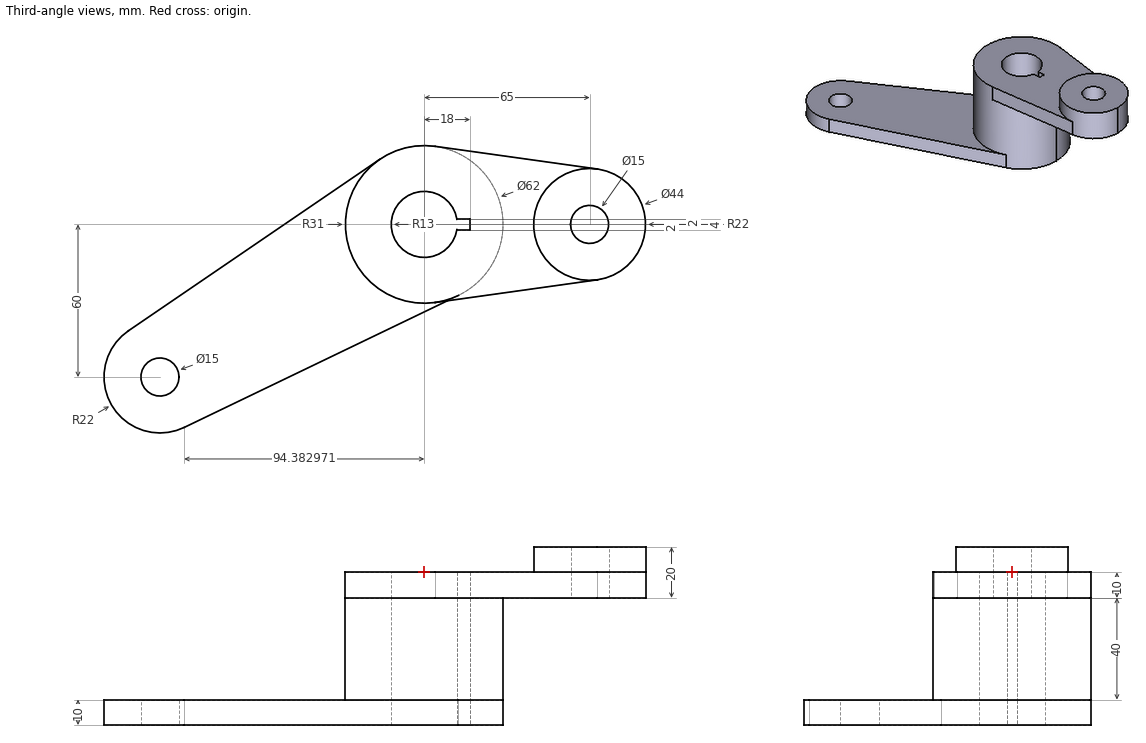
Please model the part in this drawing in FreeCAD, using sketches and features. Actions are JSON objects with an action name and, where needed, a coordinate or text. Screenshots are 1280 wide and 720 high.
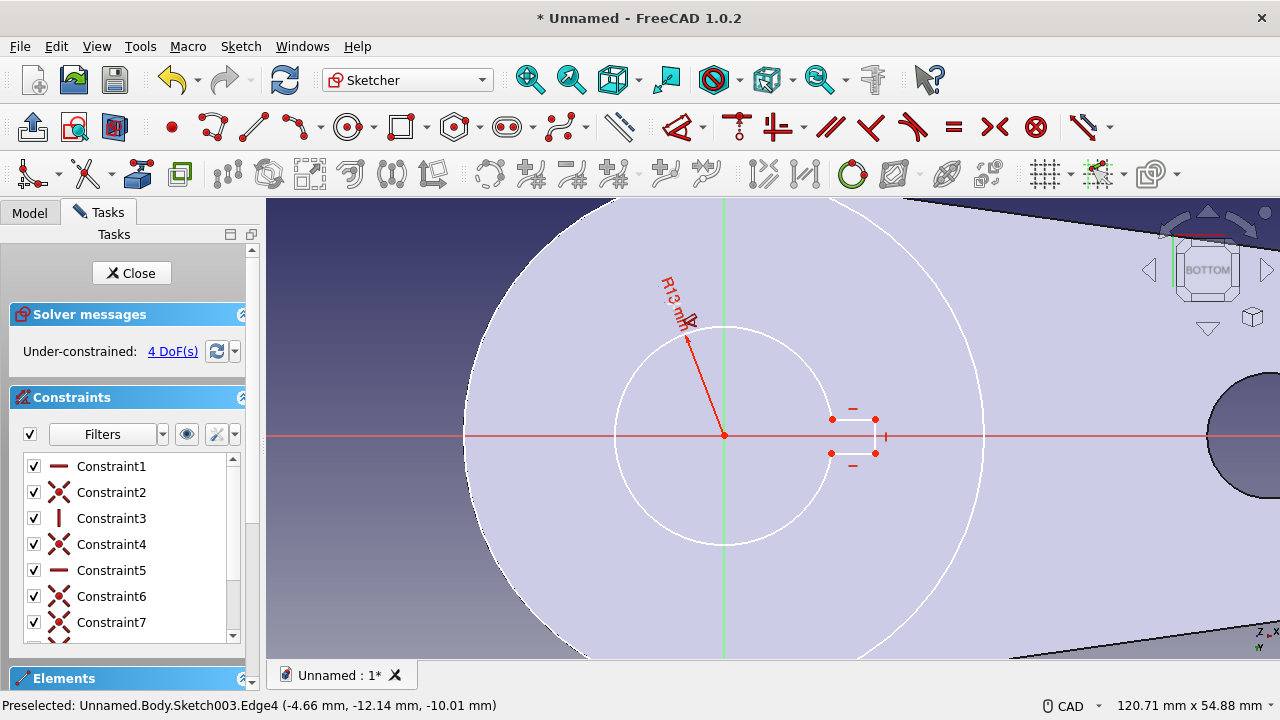
{"action": "left_click", "coordinate": [907, 251]}
{"action": "left_click", "coordinate": [930, 228]}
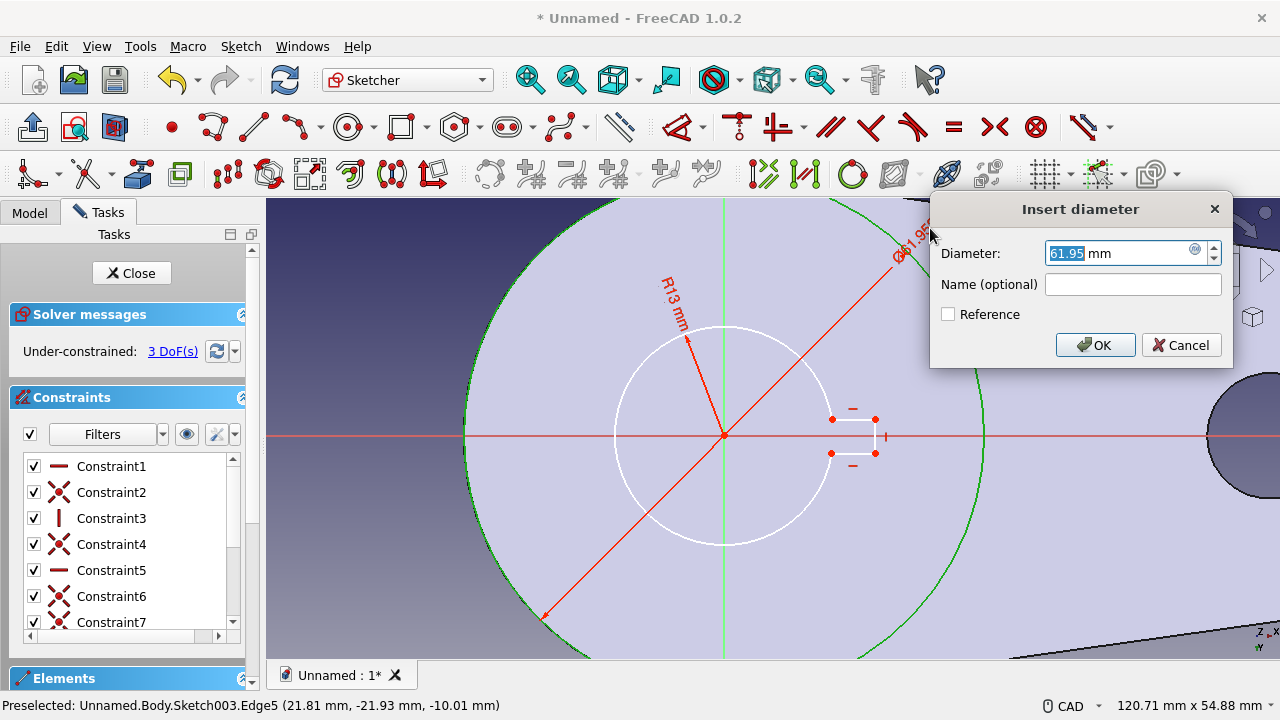
{"action": "type", "text": "62"}
{"action": "key", "text": "Return"}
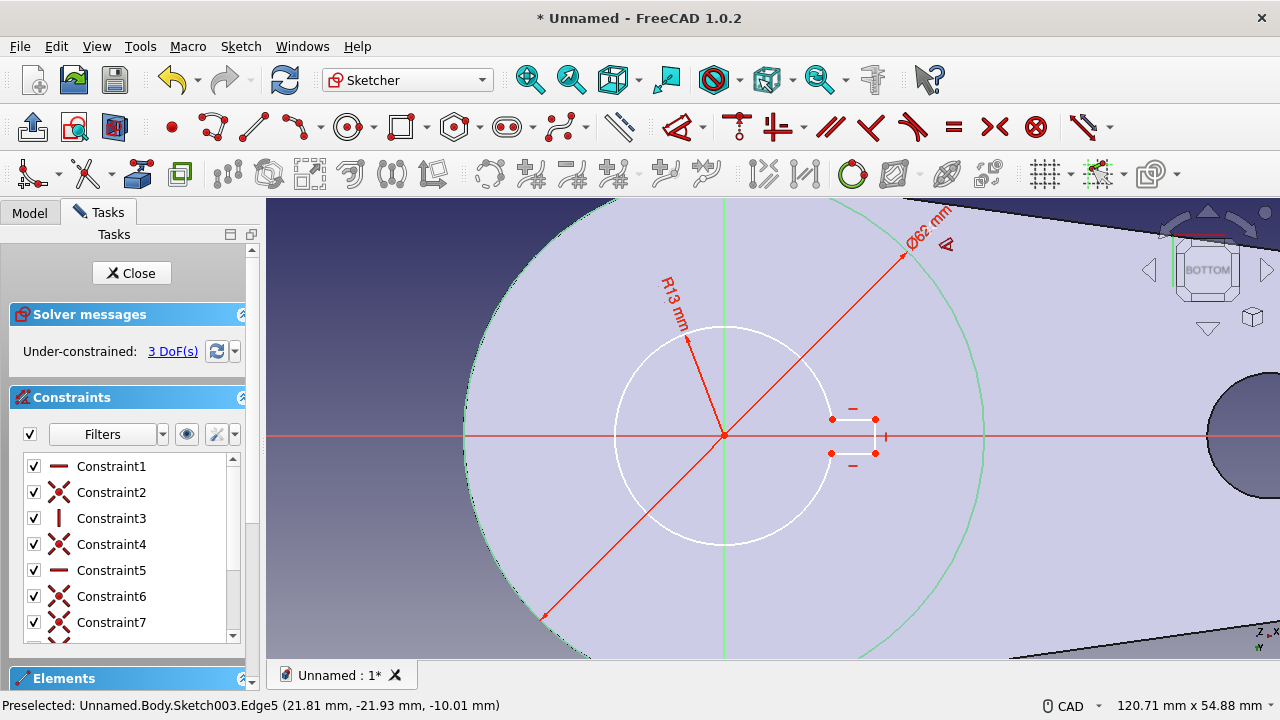
{"action": "left_click", "coordinate": [875, 434]}
{"action": "left_click", "coordinate": [909, 429]}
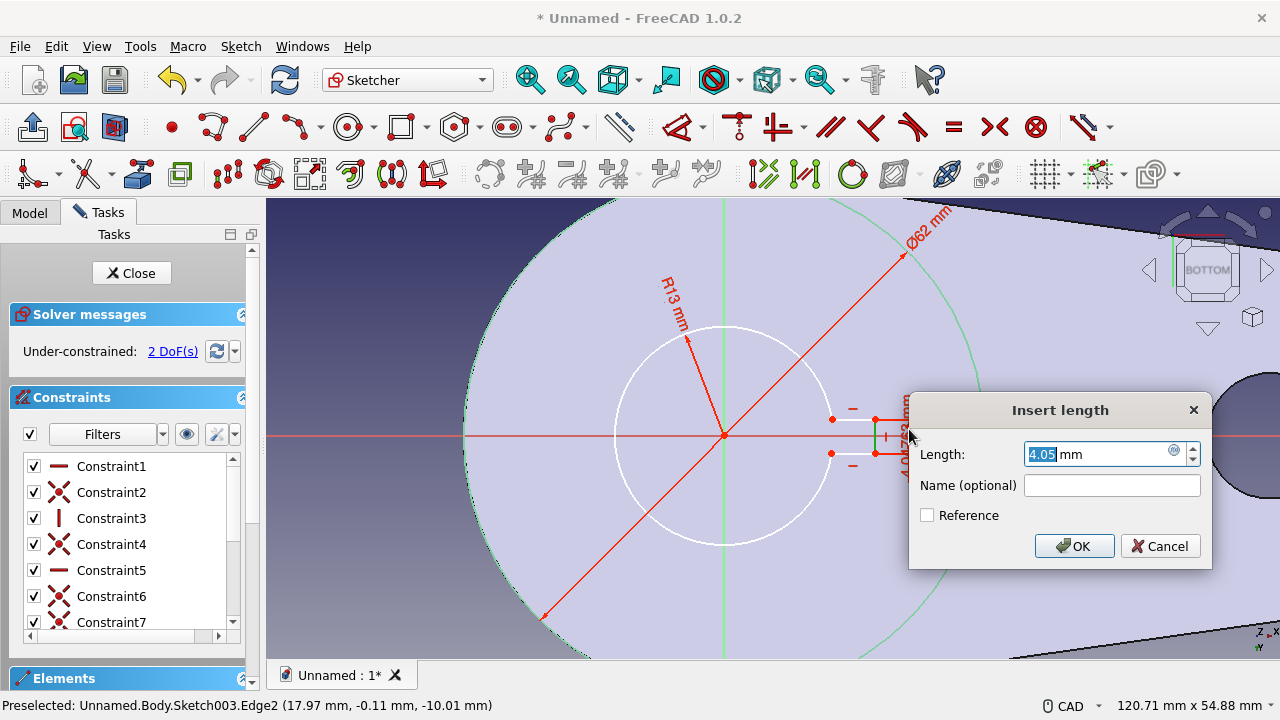
{"action": "type", "text": "4"}
{"action": "key", "text": "Return"}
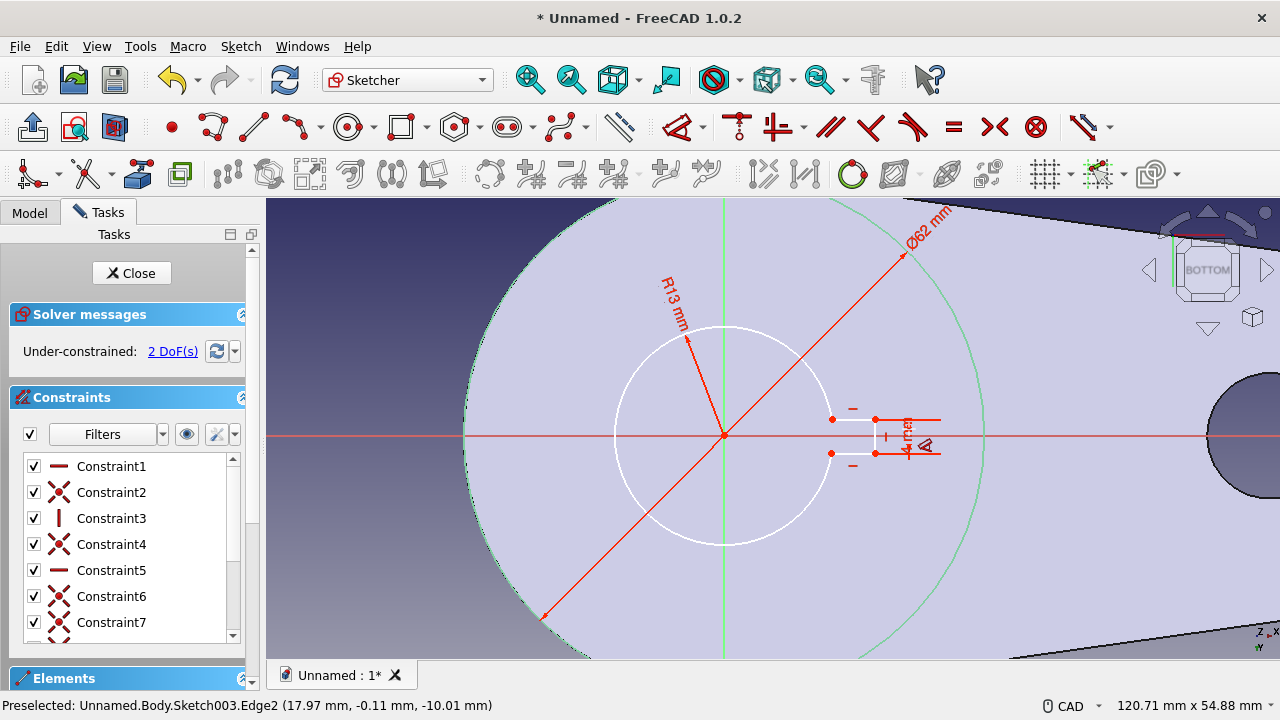
{"action": "scroll", "coordinate": [832, 420], "scroll_direction": "up", "scroll_amount": 5}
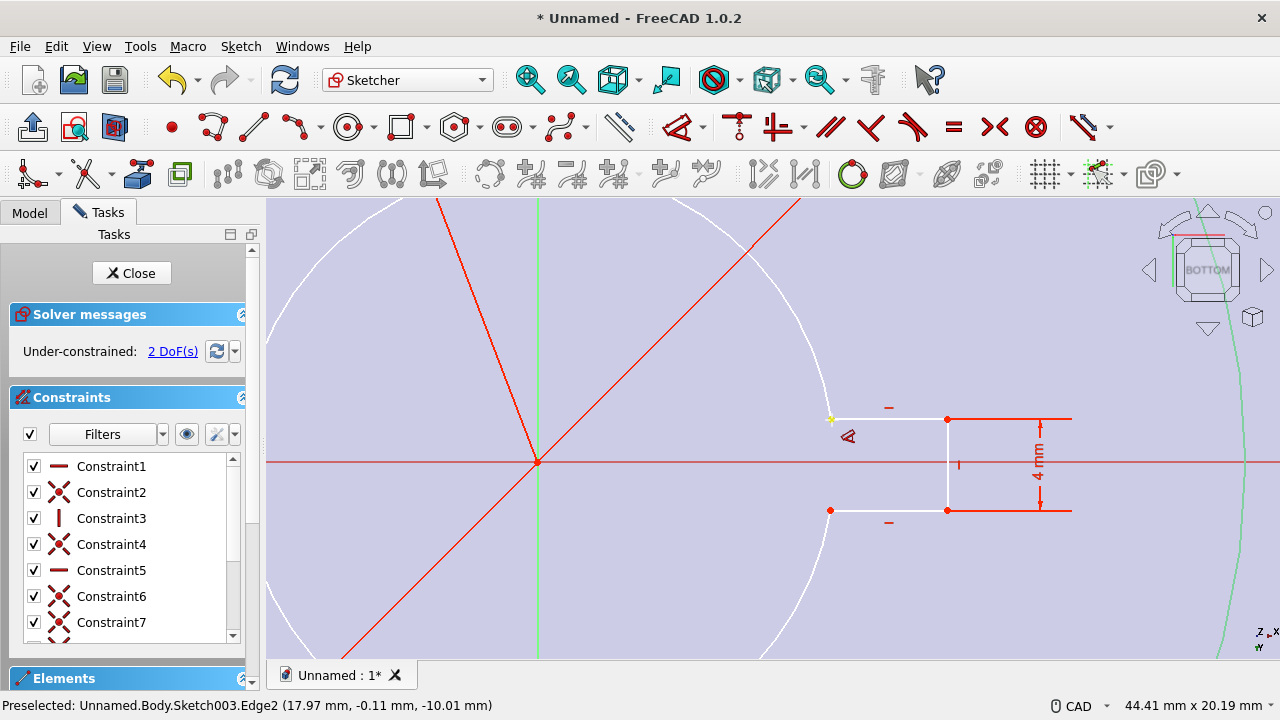
{"action": "left_click", "coordinate": [831, 419]}
{"action": "left_click", "coordinate": [865, 441]}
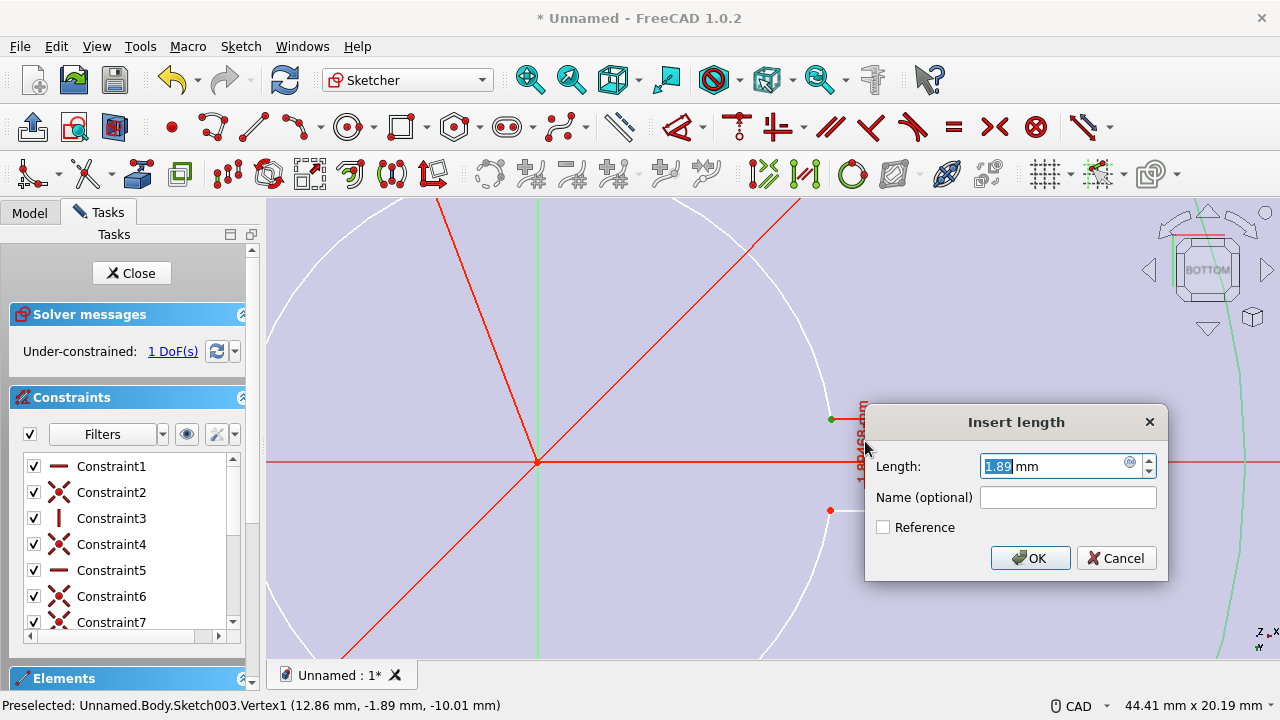
{"action": "type", "text": "2"}
{"action": "key", "text": "Return"}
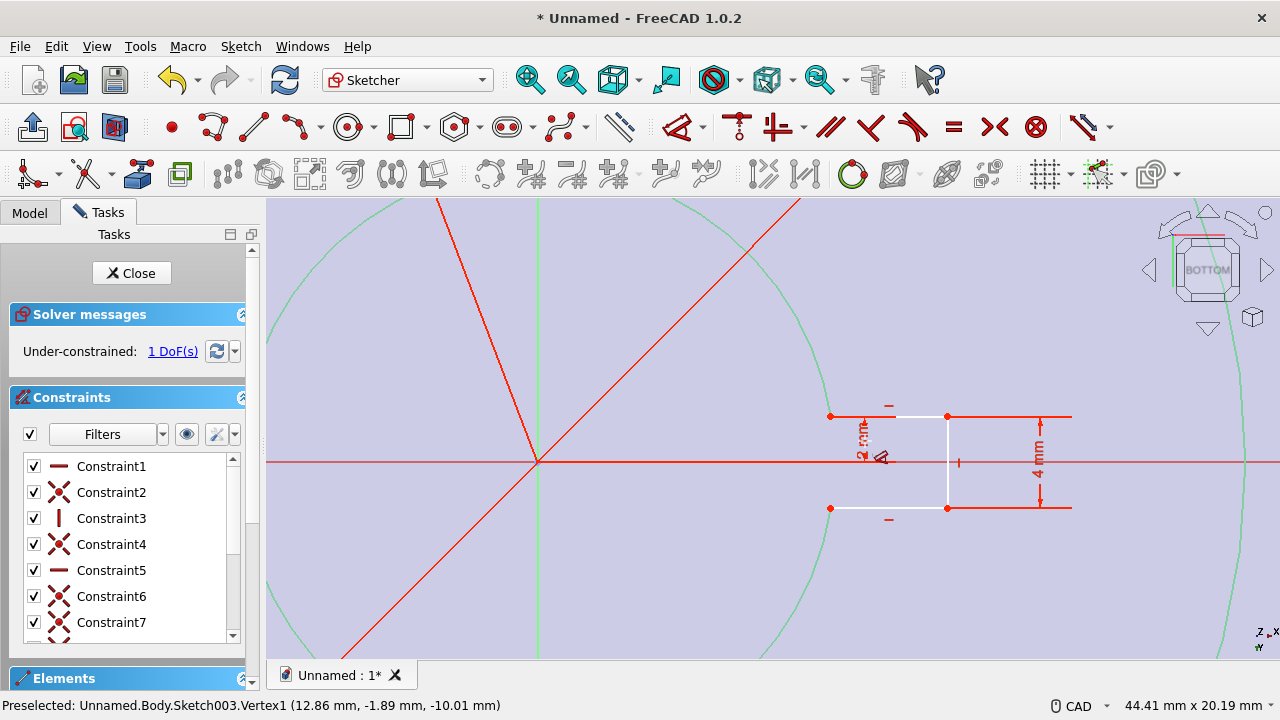
{"action": "scroll", "coordinate": [747, 420], "scroll_direction": "down", "scroll_amount": 8}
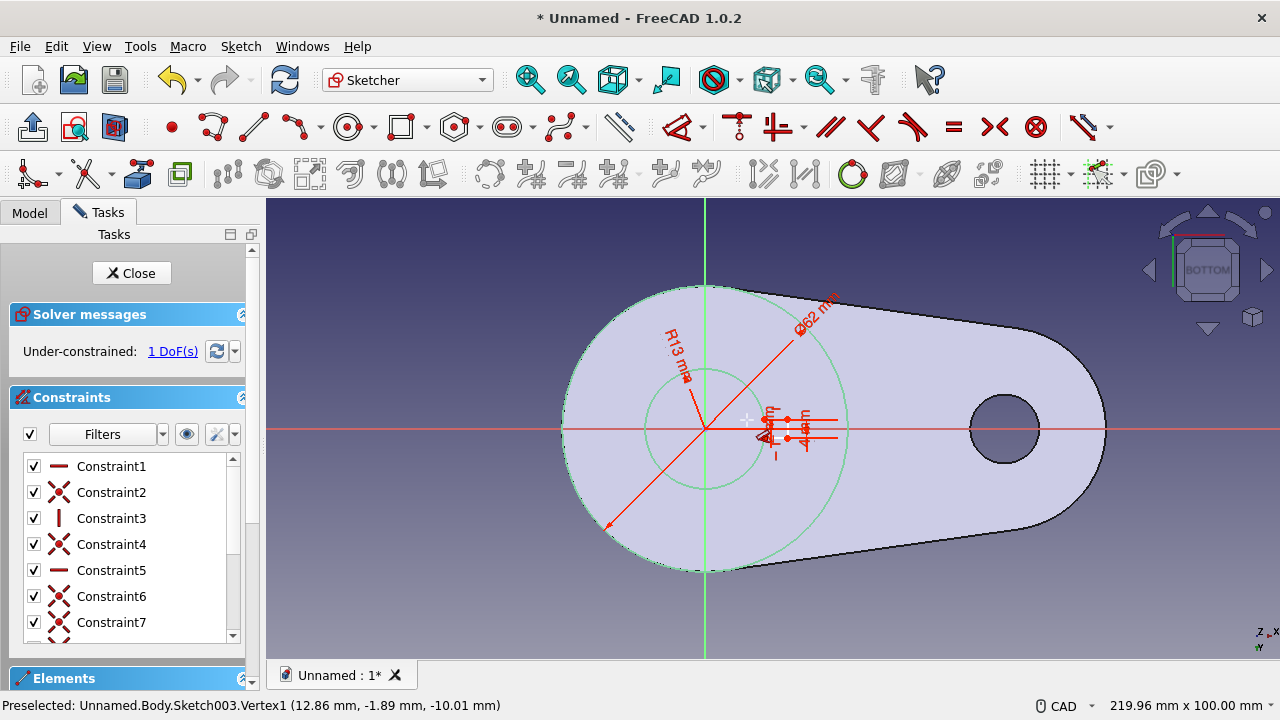
{"action": "left_click", "coordinate": [788, 420]}
{"action": "left_click", "coordinate": [766, 386]}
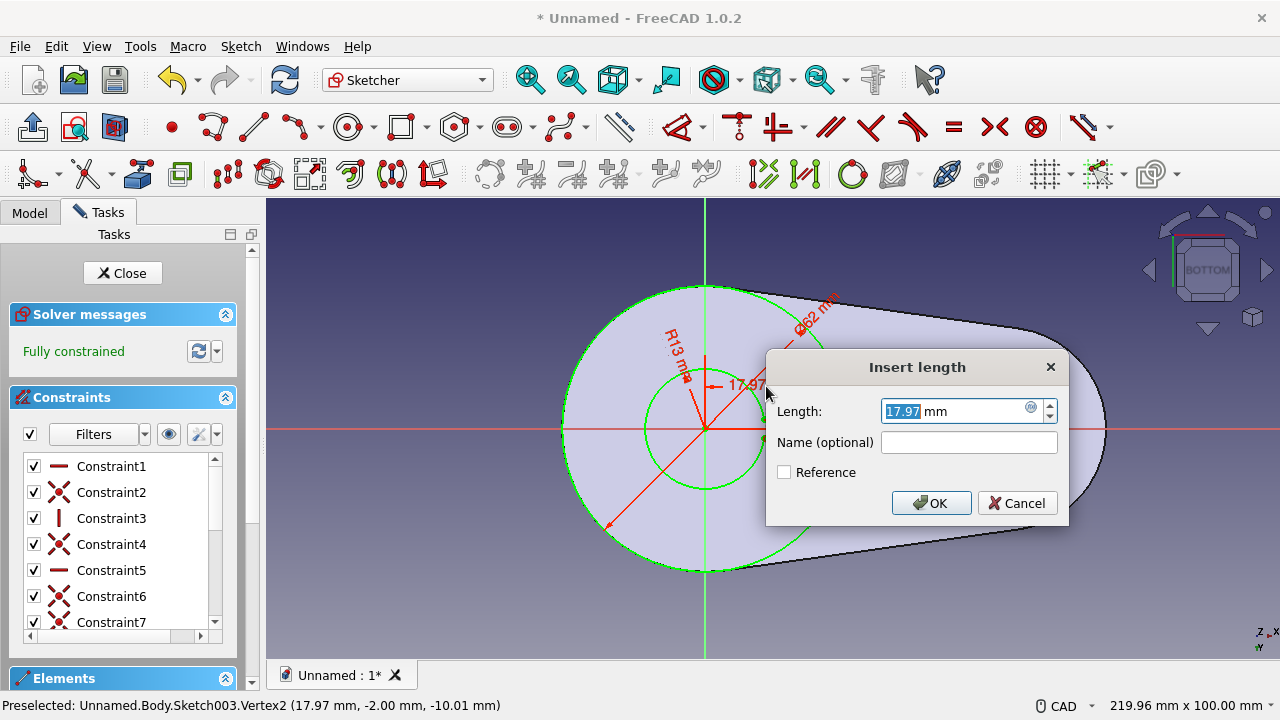
{"action": "type", "text": "18"}
{"action": "key", "text": "Return"}
{"action": "key", "text": "Escape"}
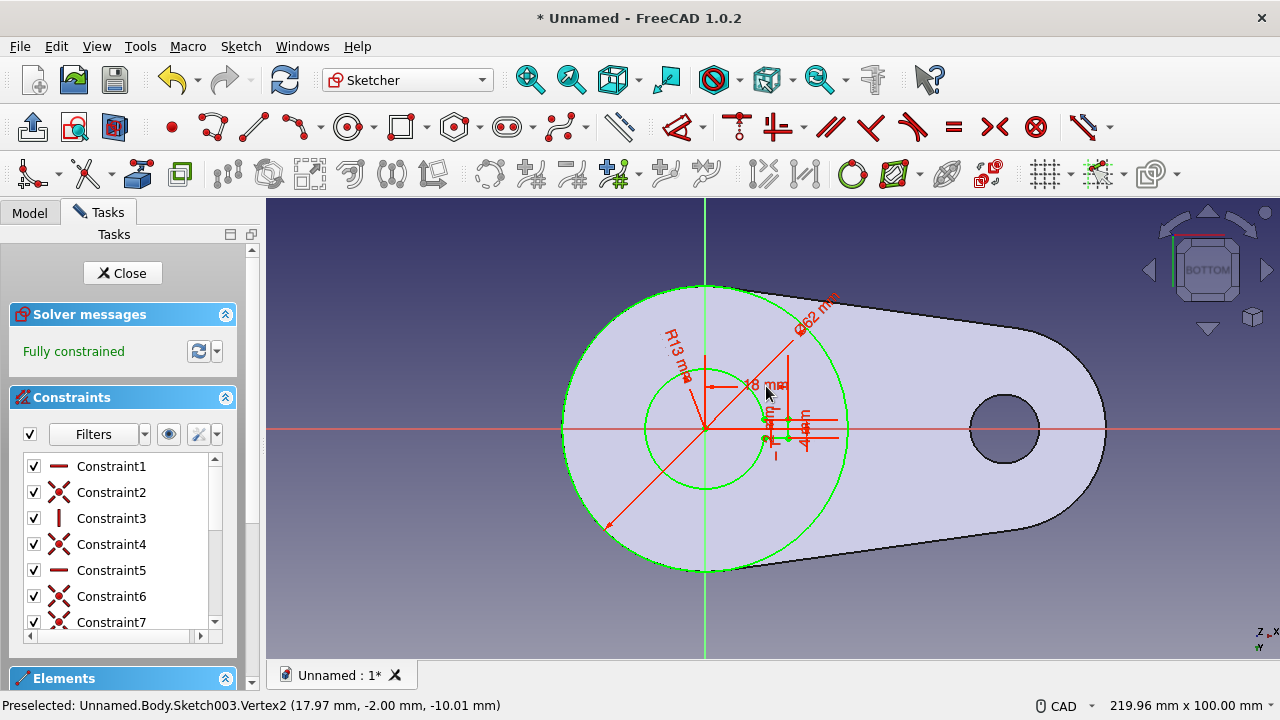
{"action": "left_click", "coordinate": [123, 273]}